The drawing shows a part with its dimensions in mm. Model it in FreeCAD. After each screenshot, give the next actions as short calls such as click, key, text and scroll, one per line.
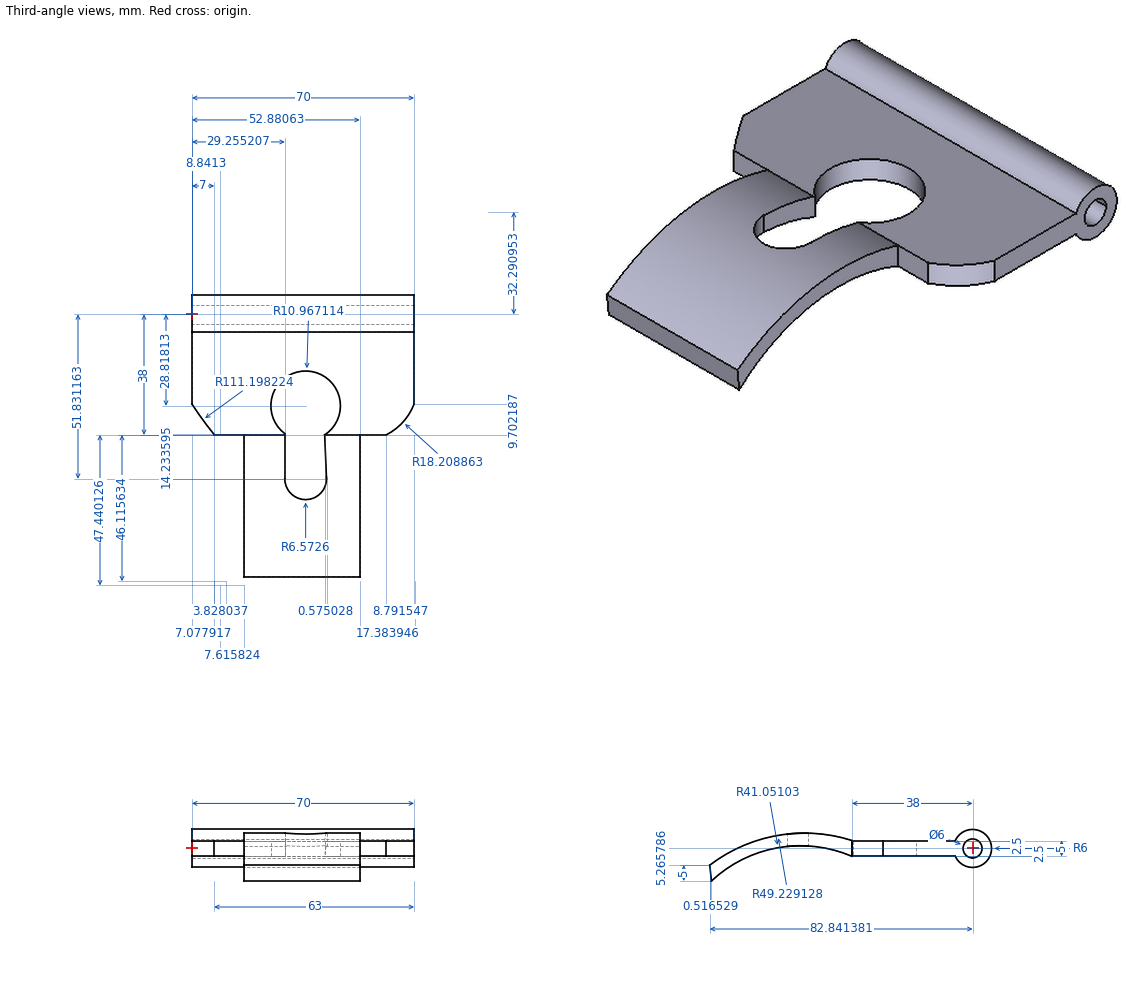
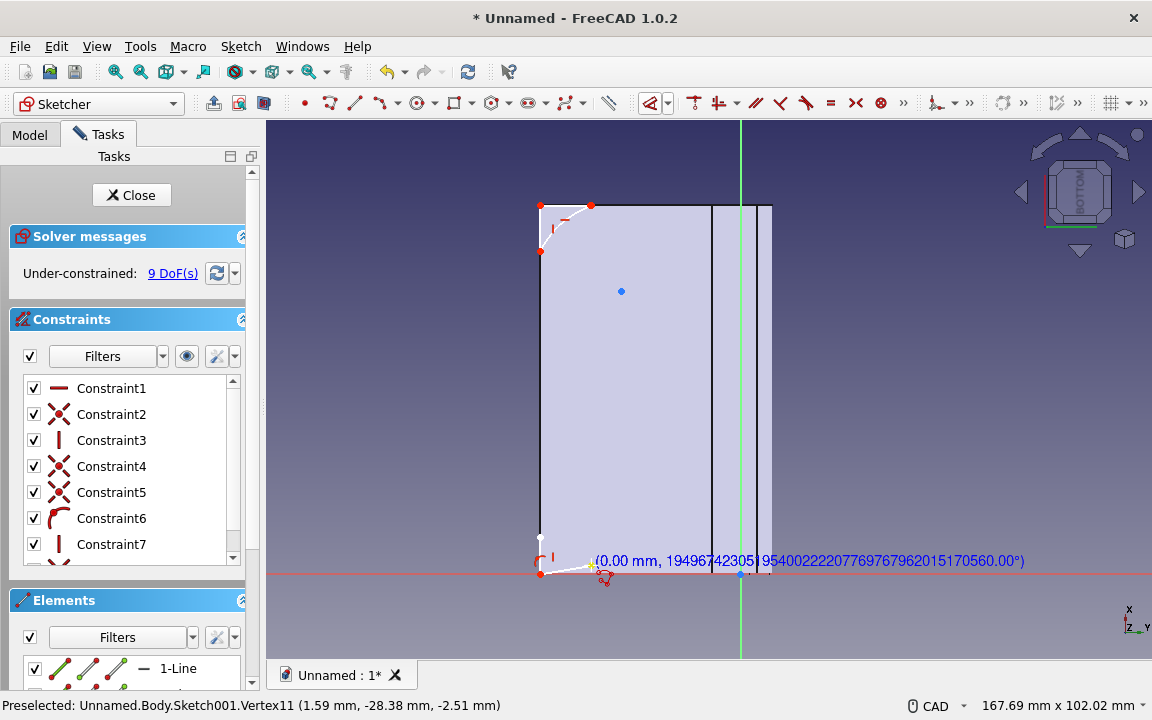
click(380, 104)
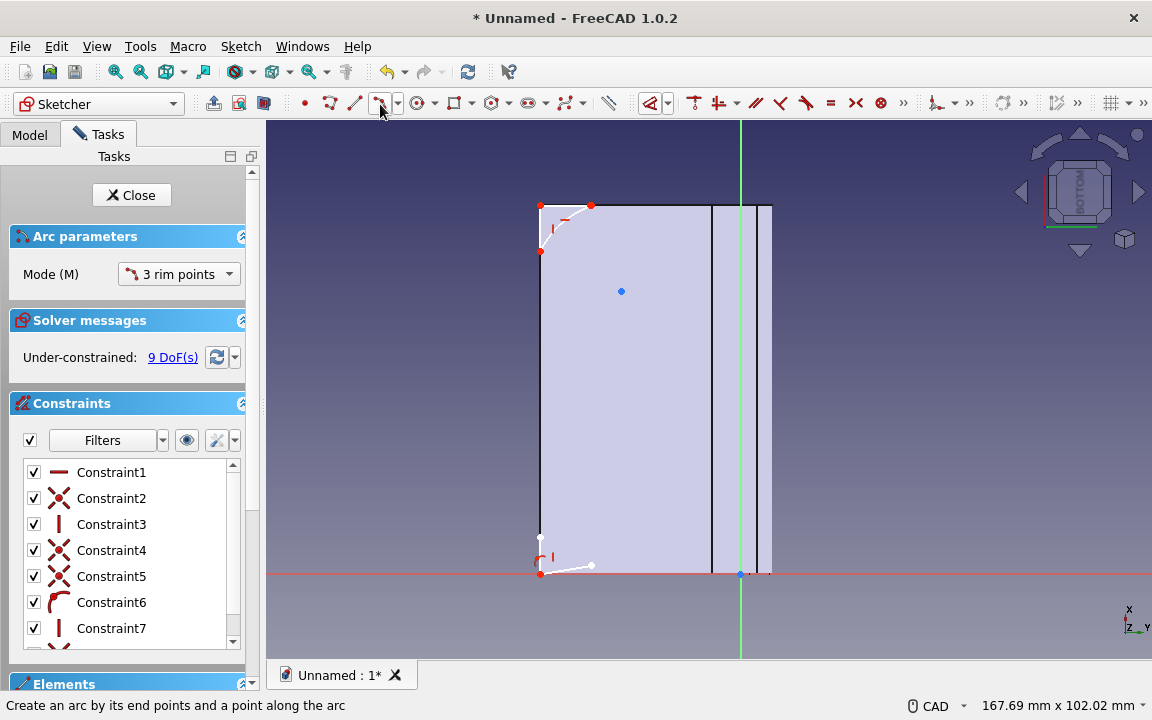
click(591, 566)
click(540, 538)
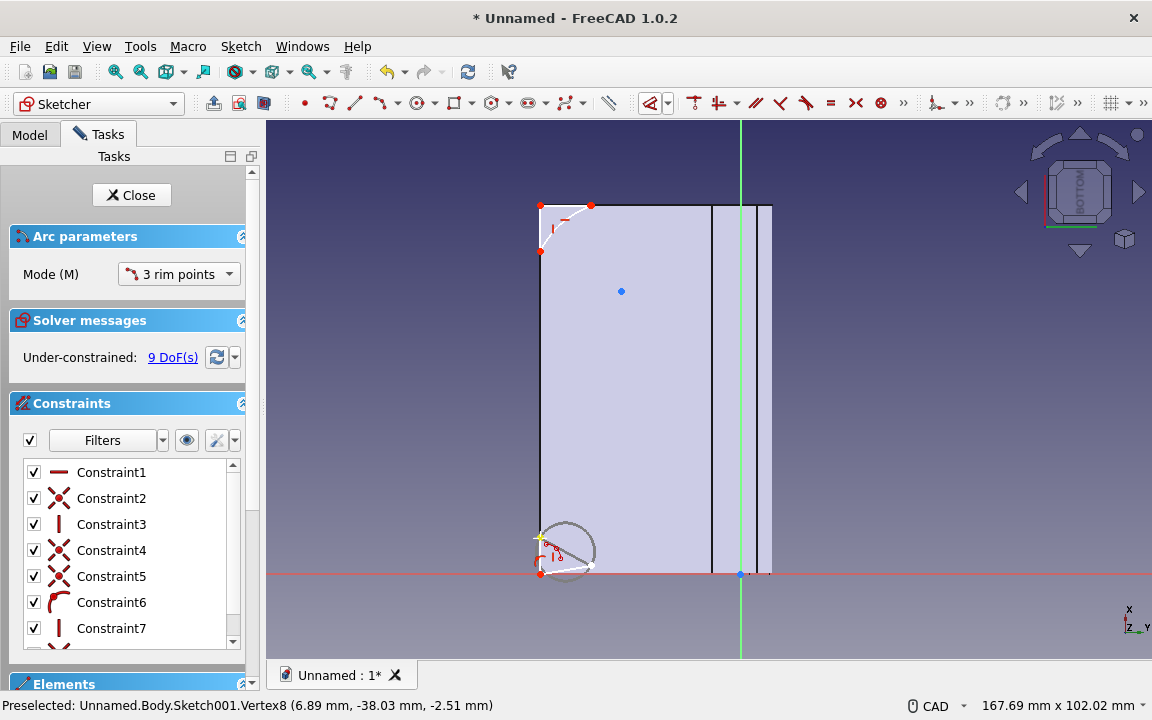
scroll(565, 556, up, 15)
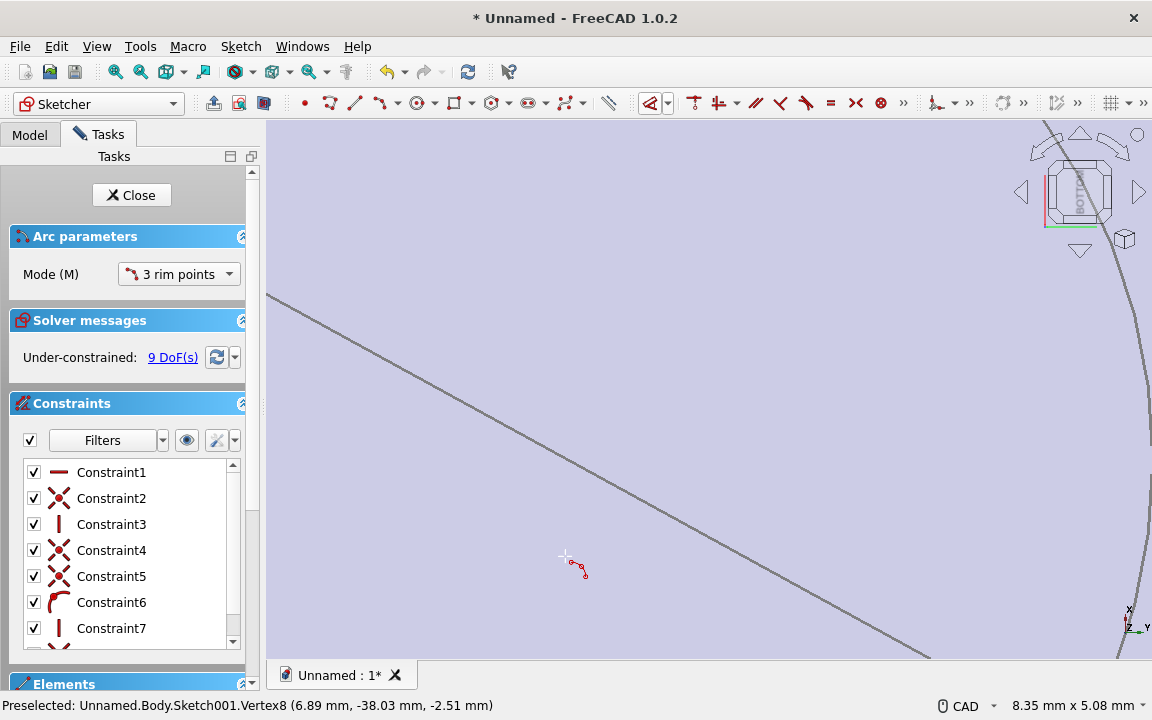
click(564, 549)
key(Escape)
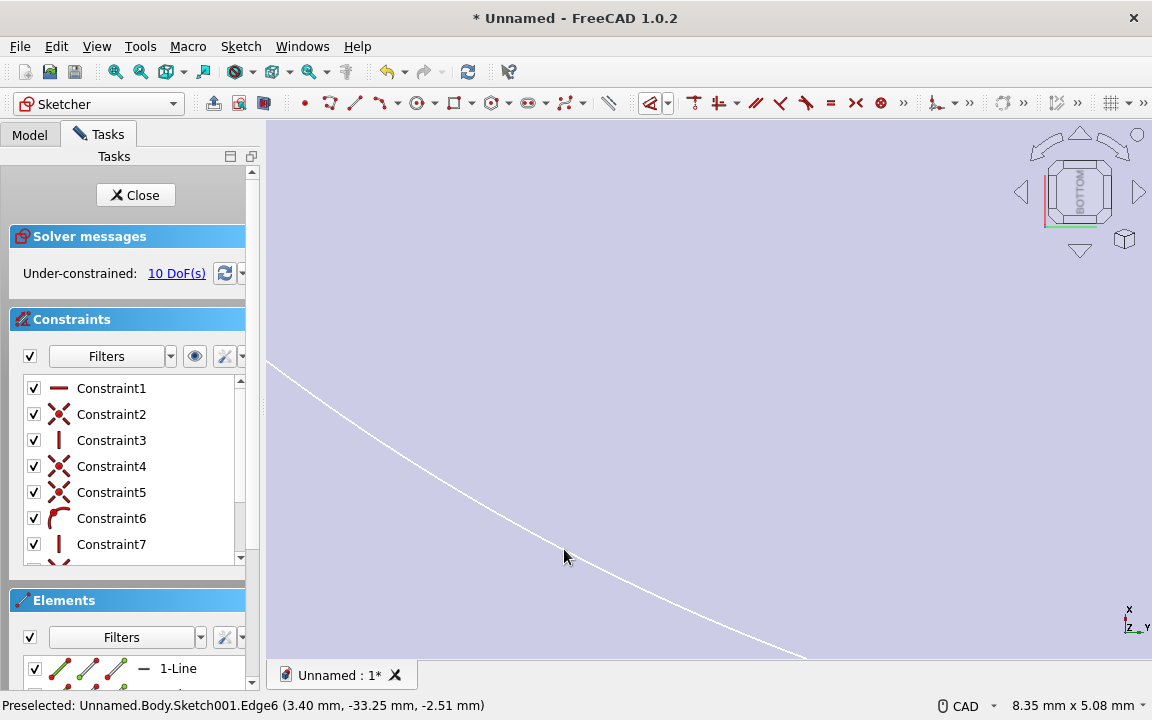
scroll(565, 557, down, 15)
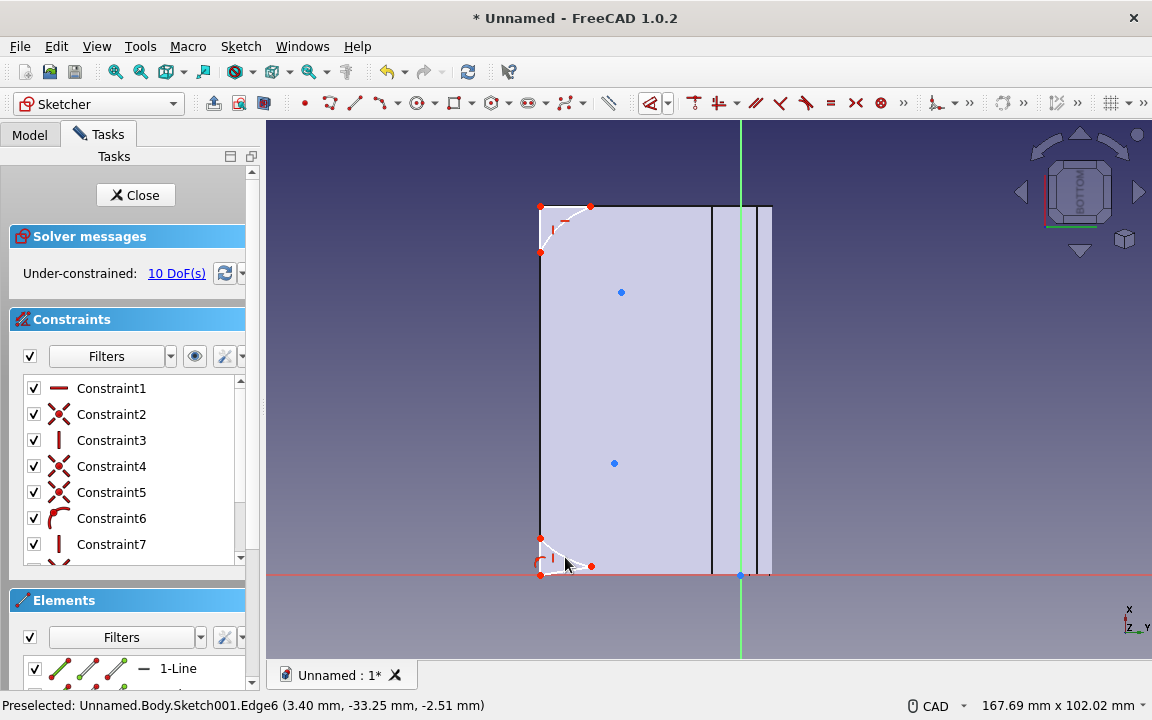
scroll(555, 573, up, 9)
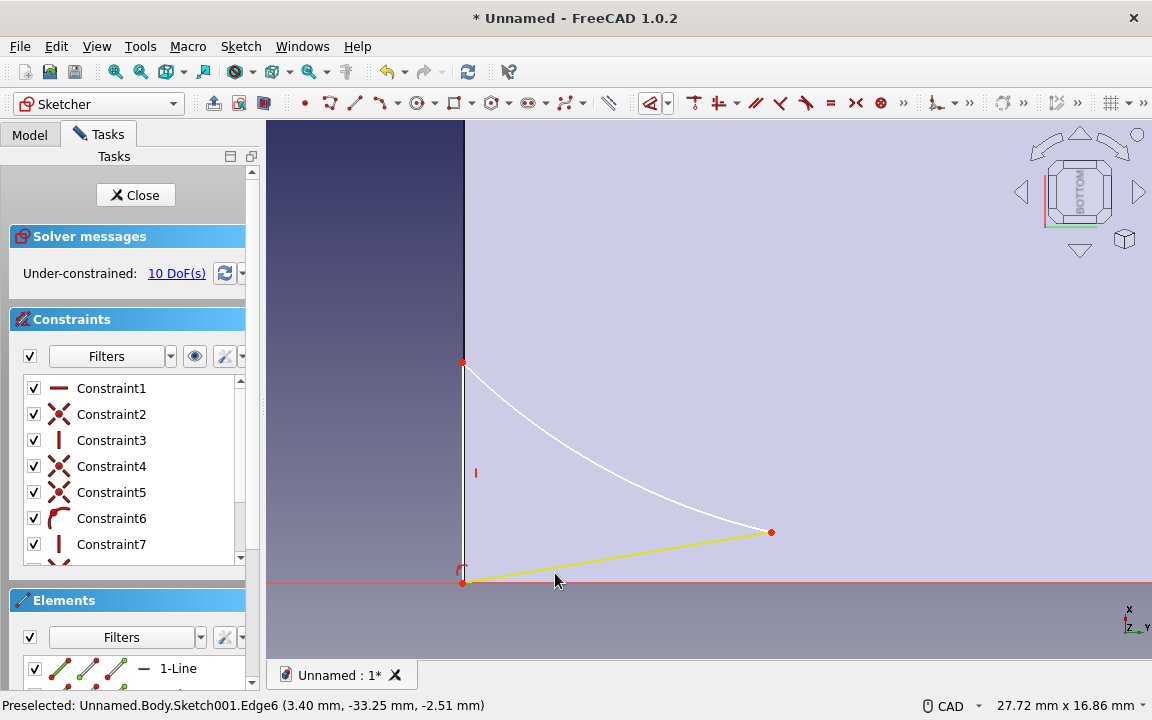
click(555, 568)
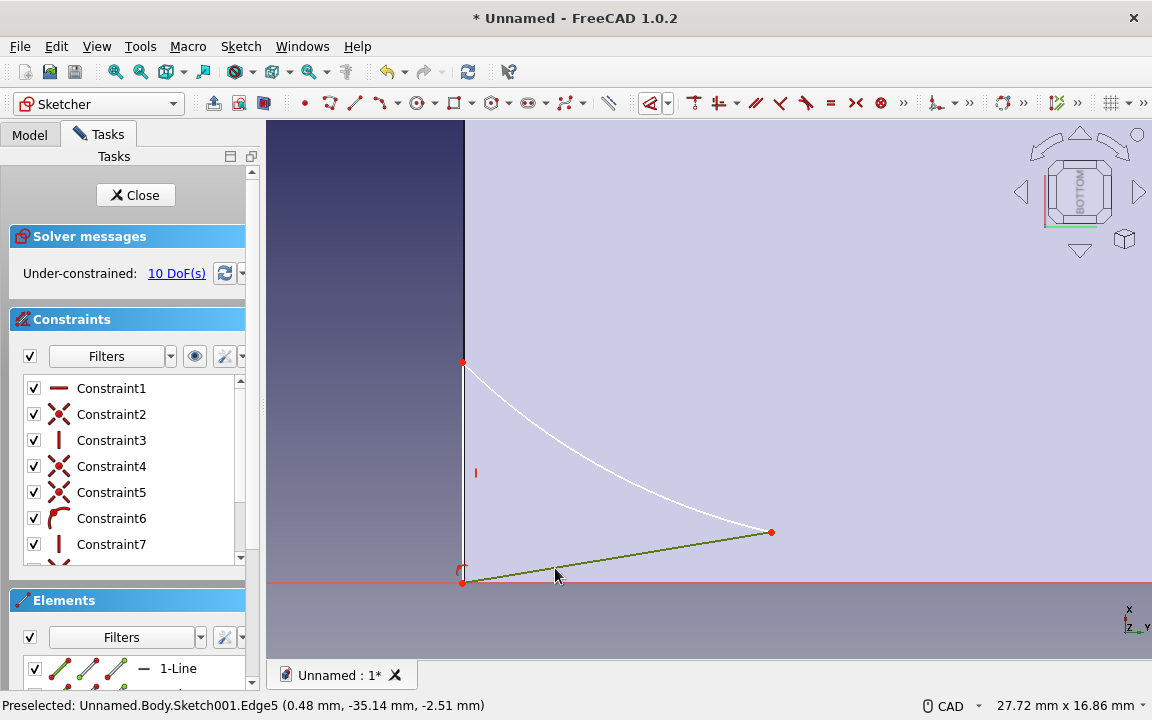
key(h)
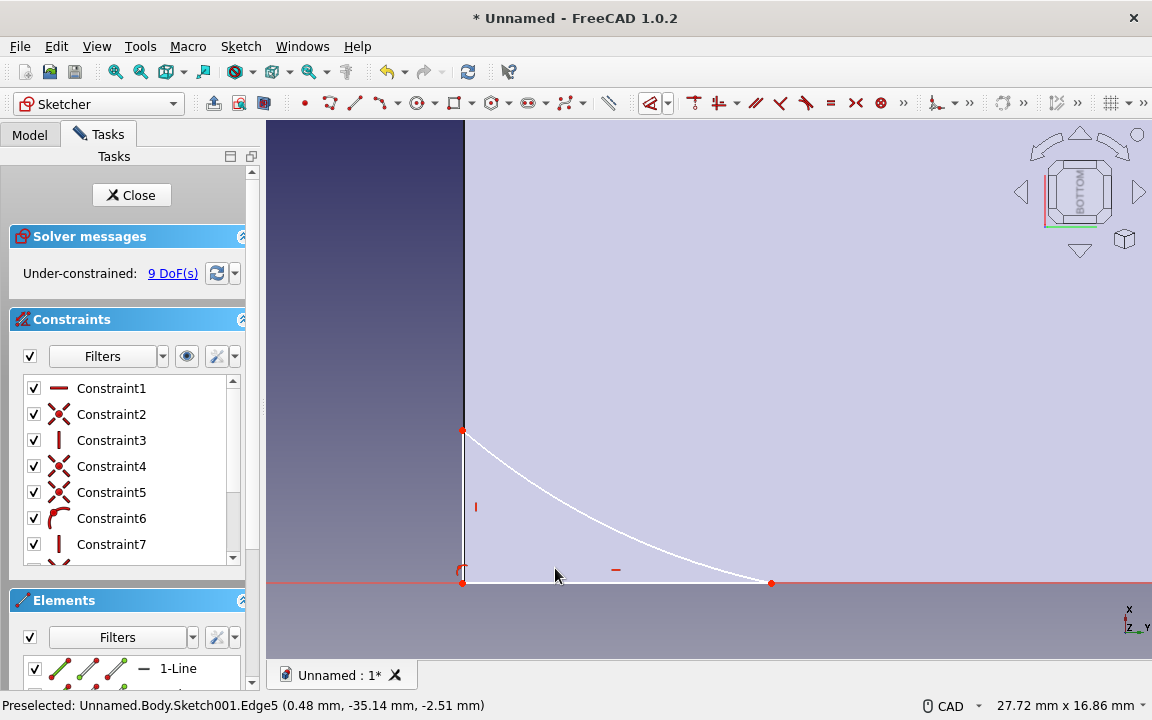
scroll(555, 573, down, 9)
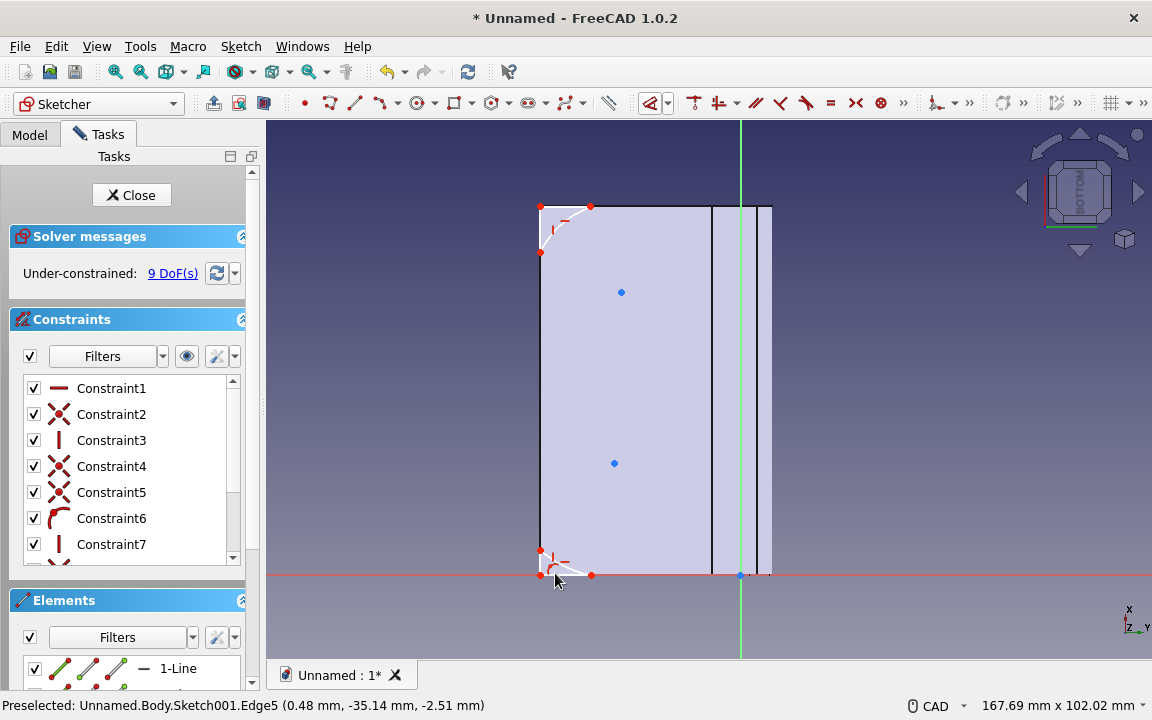
scroll(572, 216, up, 2)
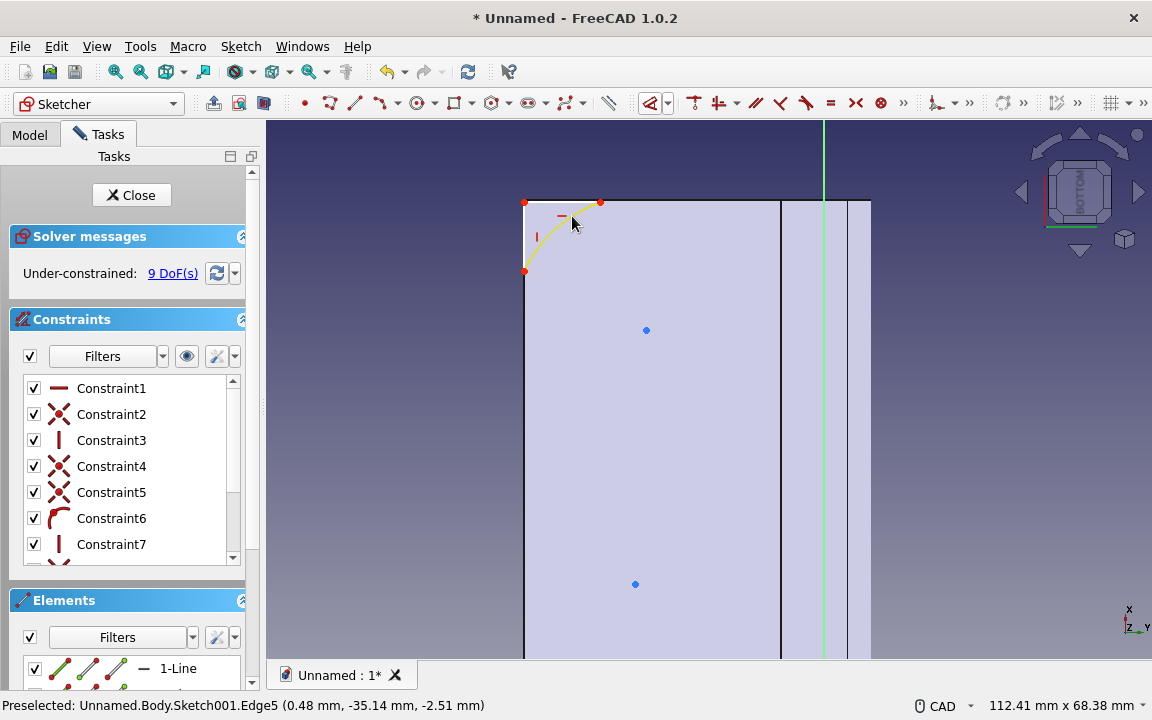
click(572, 216)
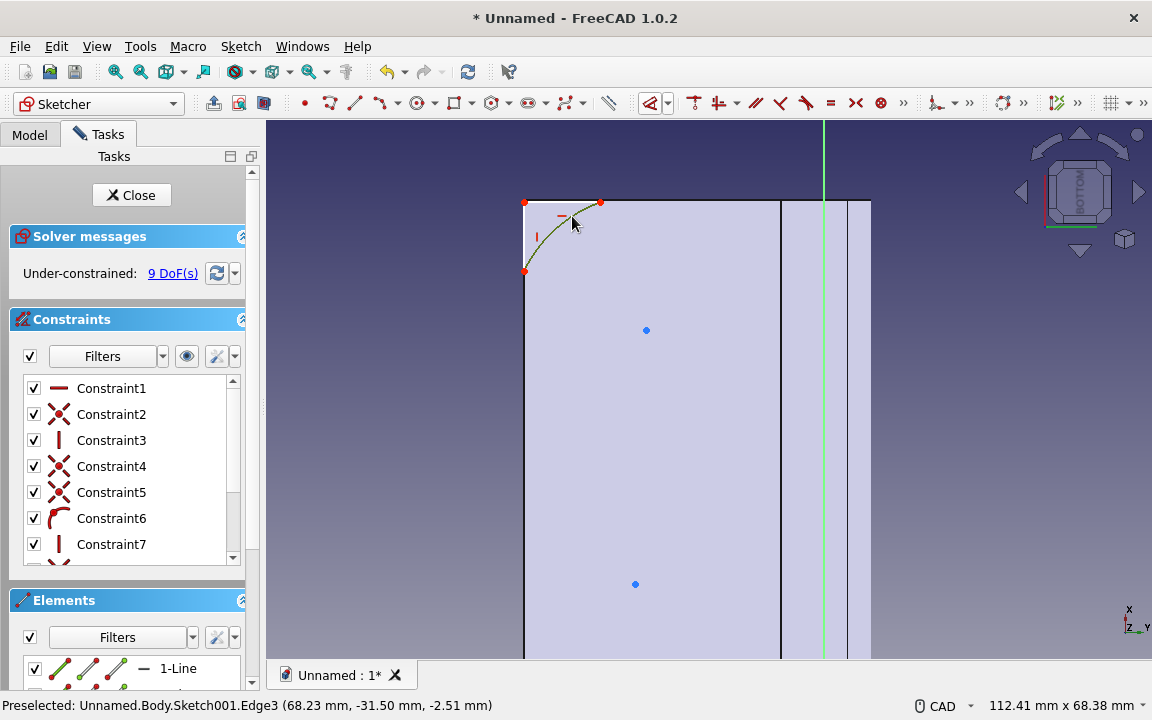
key(k)
key(r)